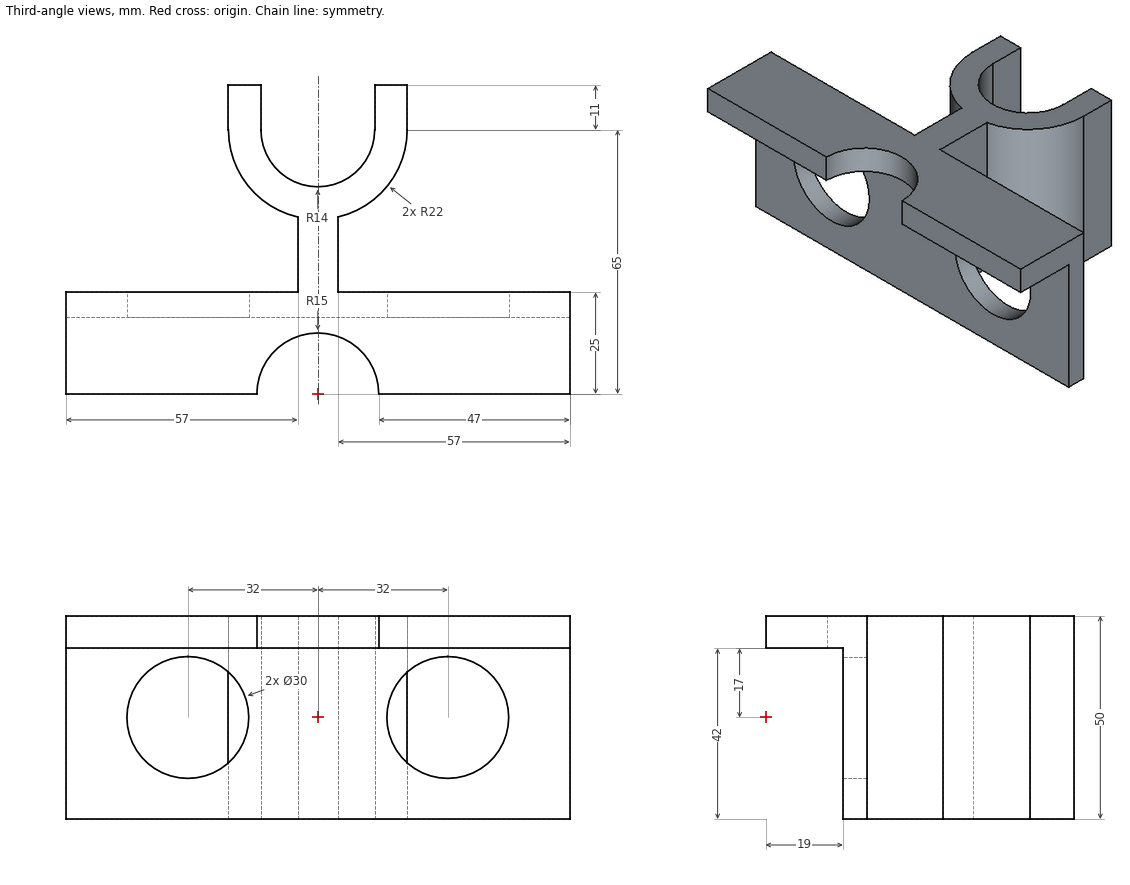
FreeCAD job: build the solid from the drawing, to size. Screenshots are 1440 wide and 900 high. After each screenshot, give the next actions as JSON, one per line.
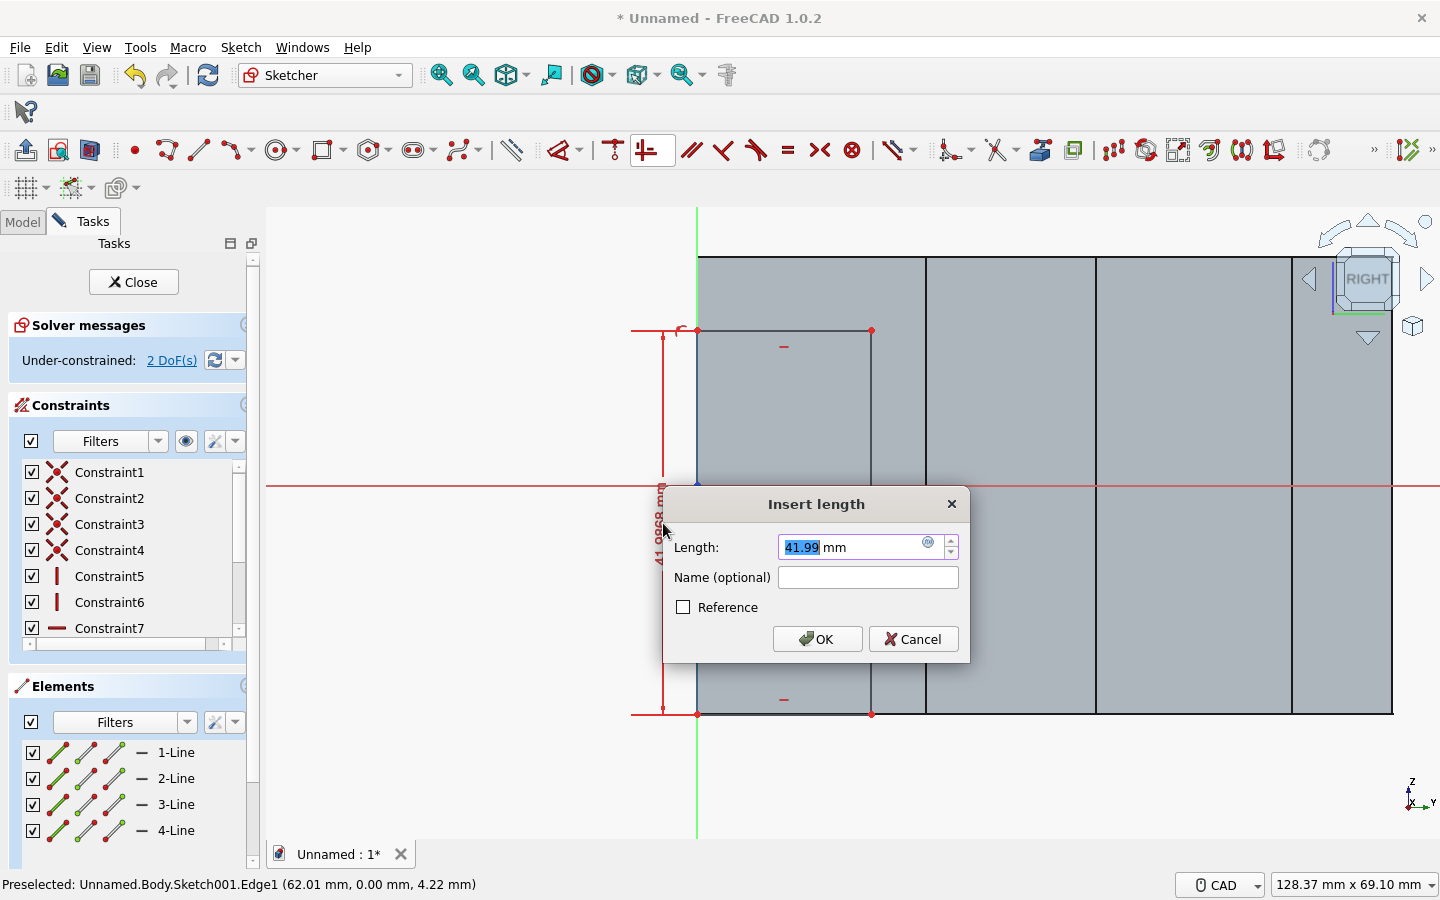
{"action": "type", "text": "42"}
{"action": "key", "text": "Return"}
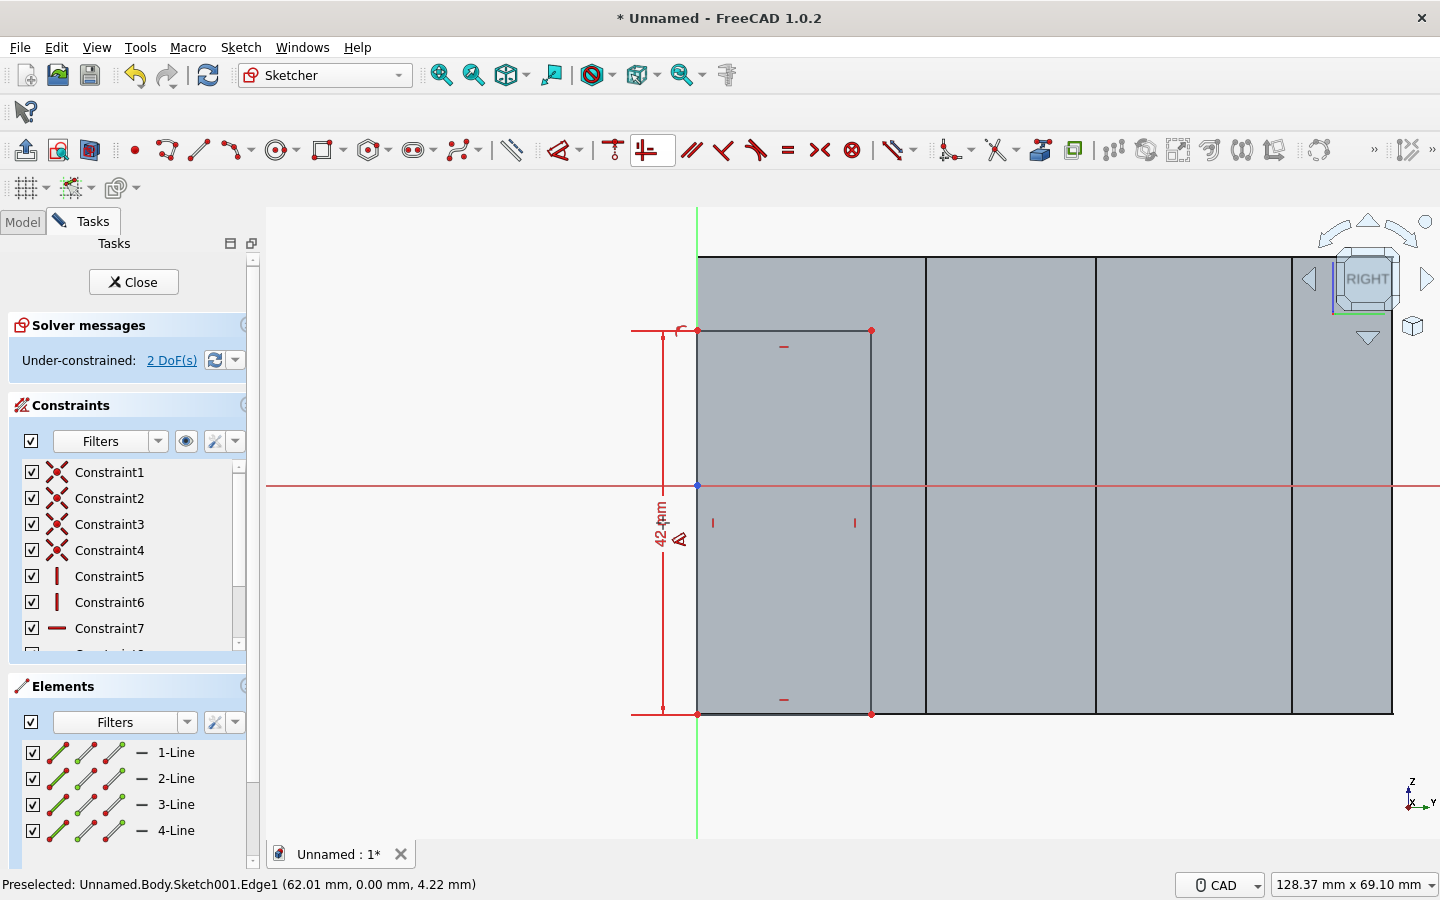
{"action": "left_click", "coordinate": [749, 715]}
{"action": "left_click", "coordinate": [784, 749]}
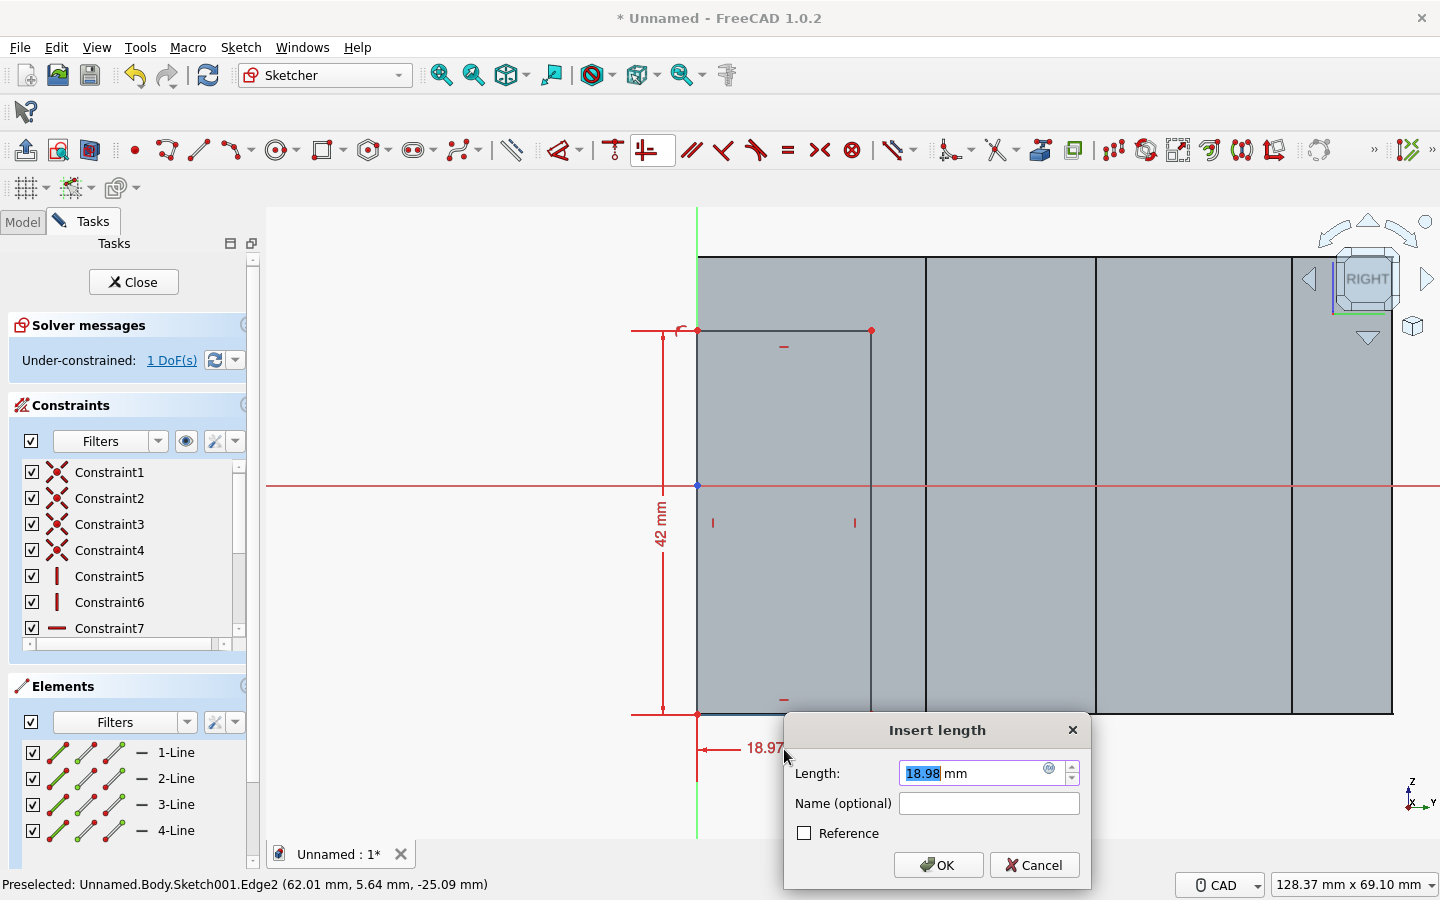
{"action": "type", "text": "19"}
{"action": "key", "text": "Return"}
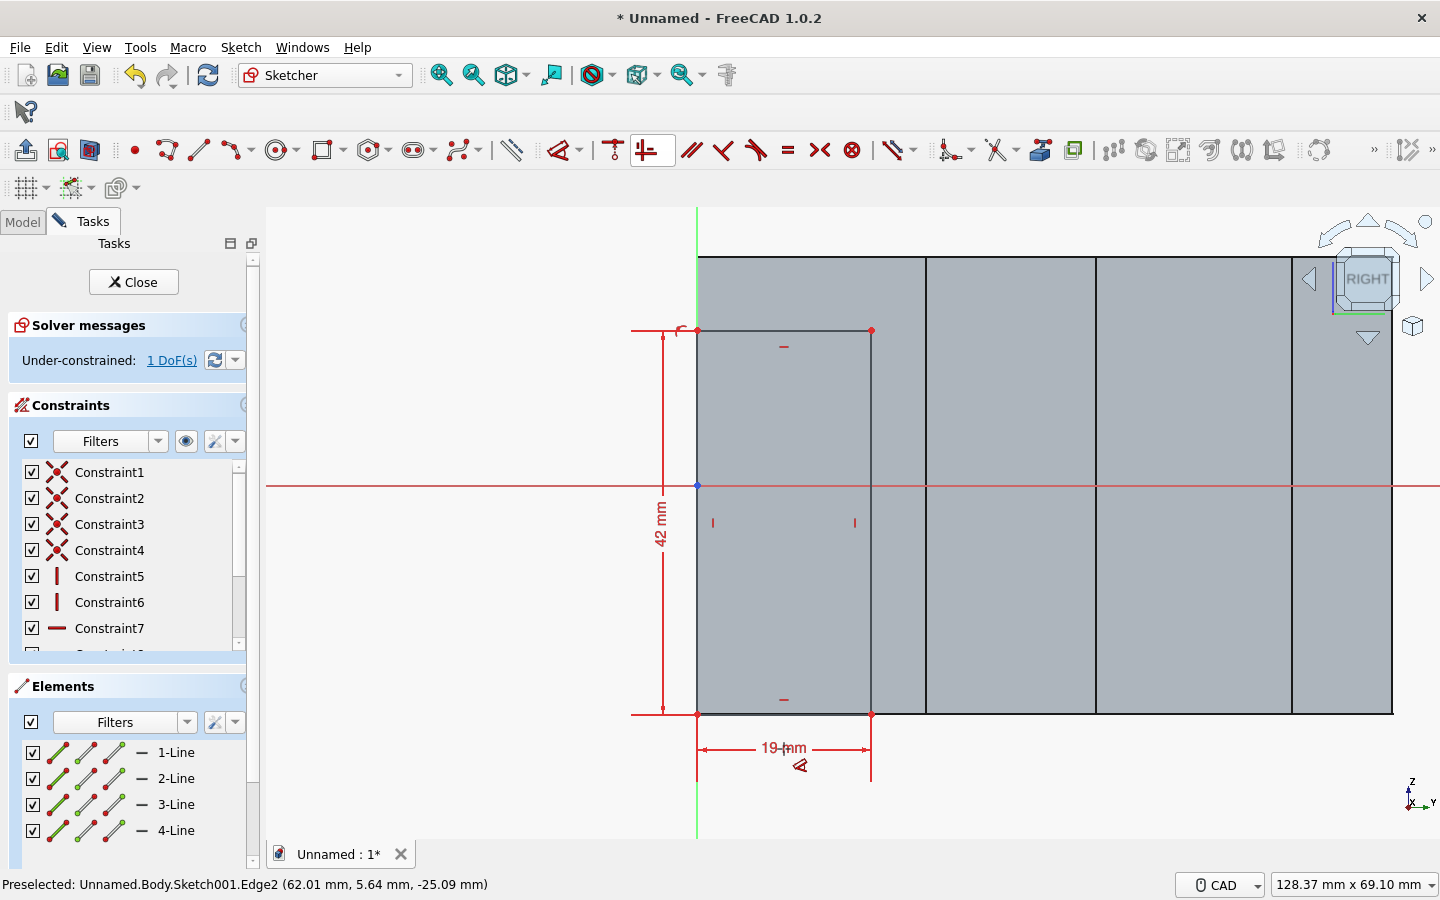
{"action": "left_click", "coordinate": [697, 331]}
{"action": "left_click", "coordinate": [663, 408]}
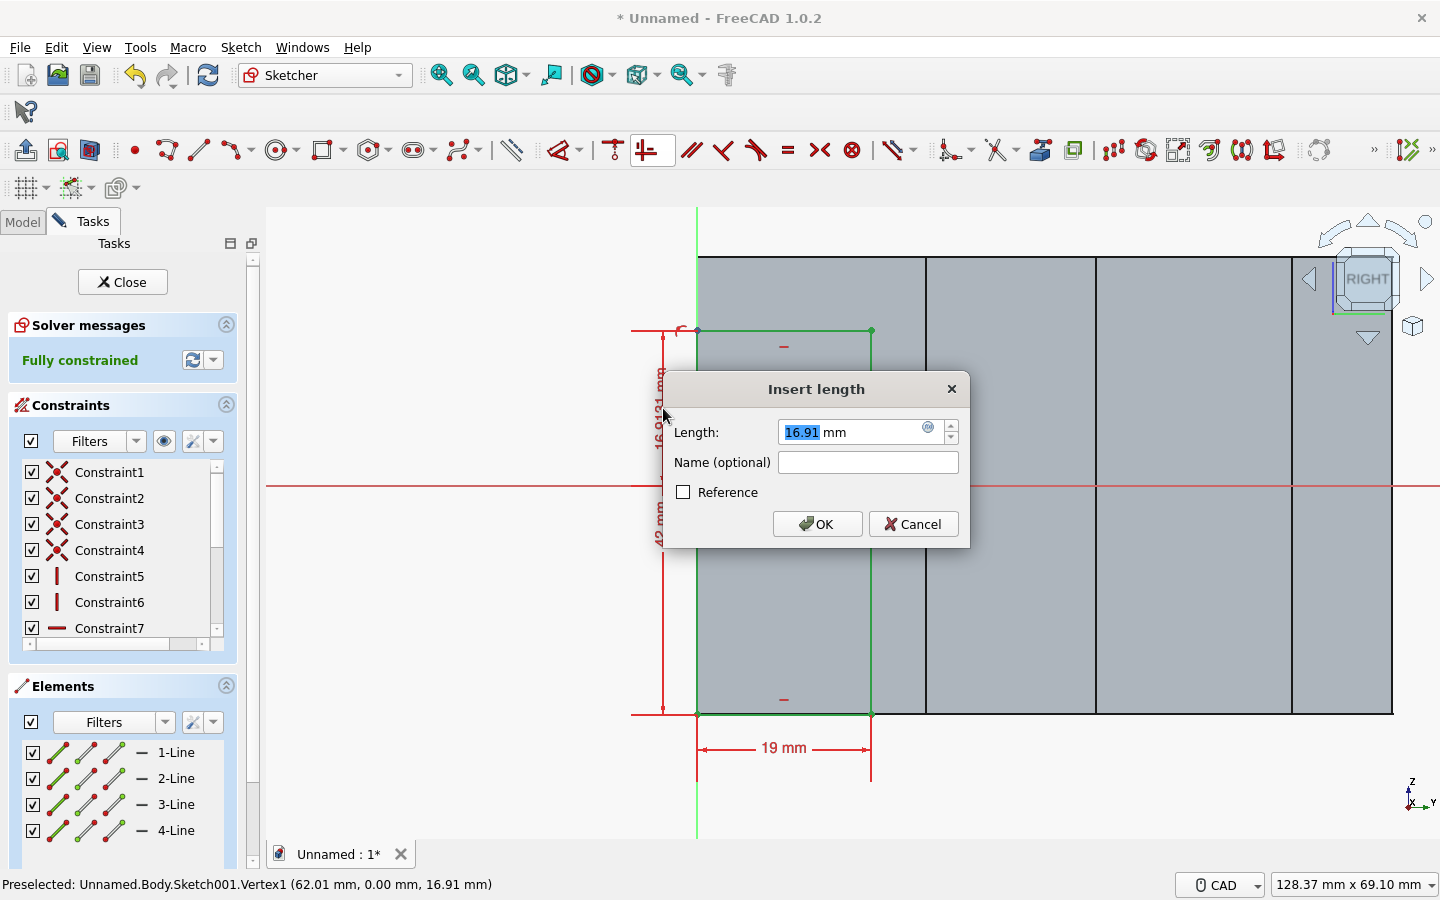
{"action": "type", "text": "17"}
{"action": "key", "text": "Return"}
{"action": "key", "text": "Escape"}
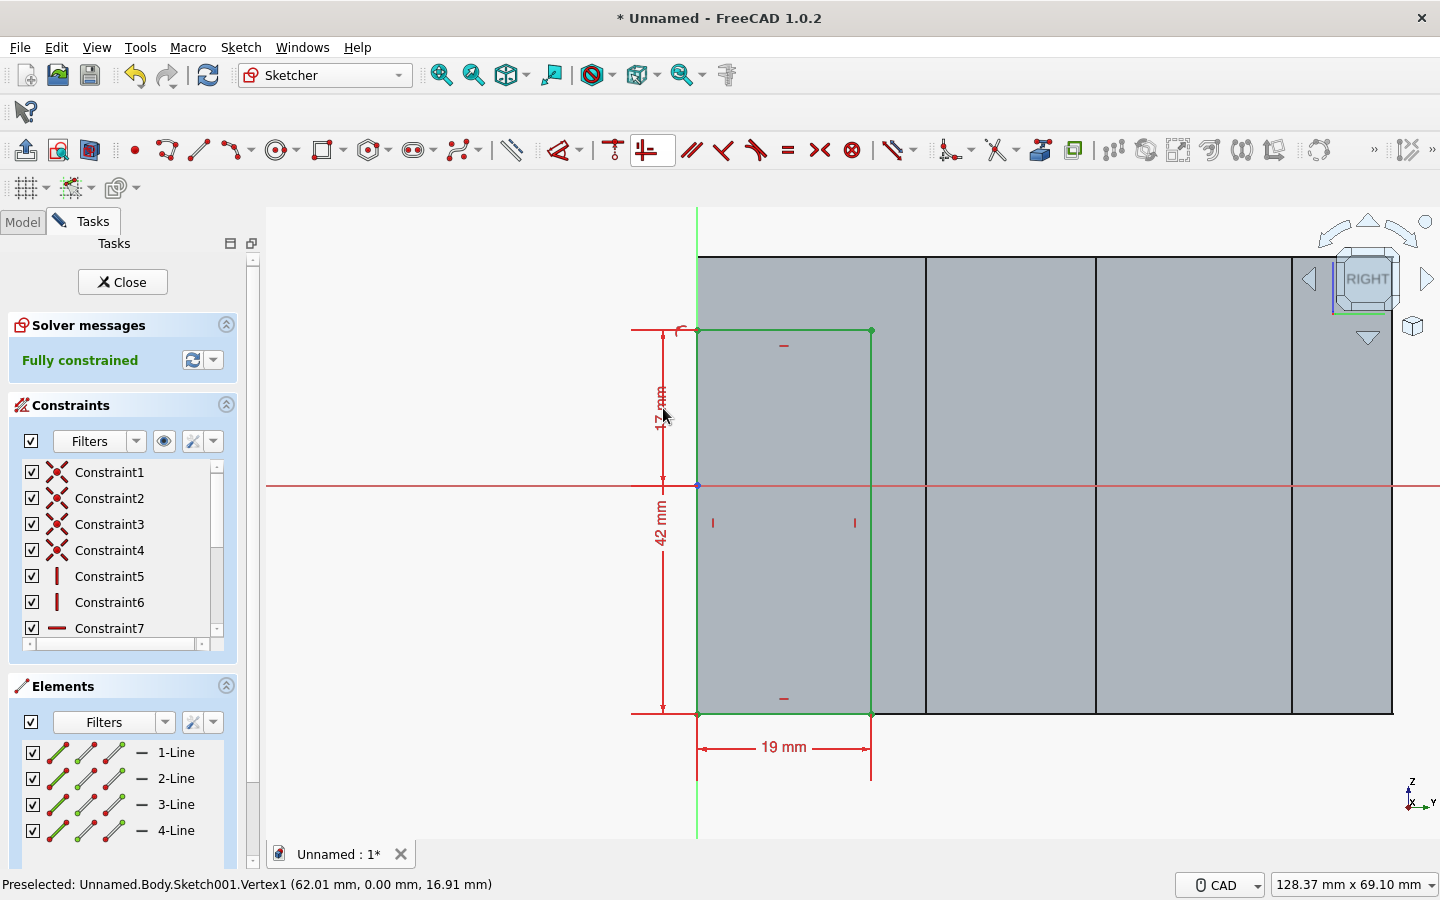
{"action": "left_click", "coordinate": [123, 282]}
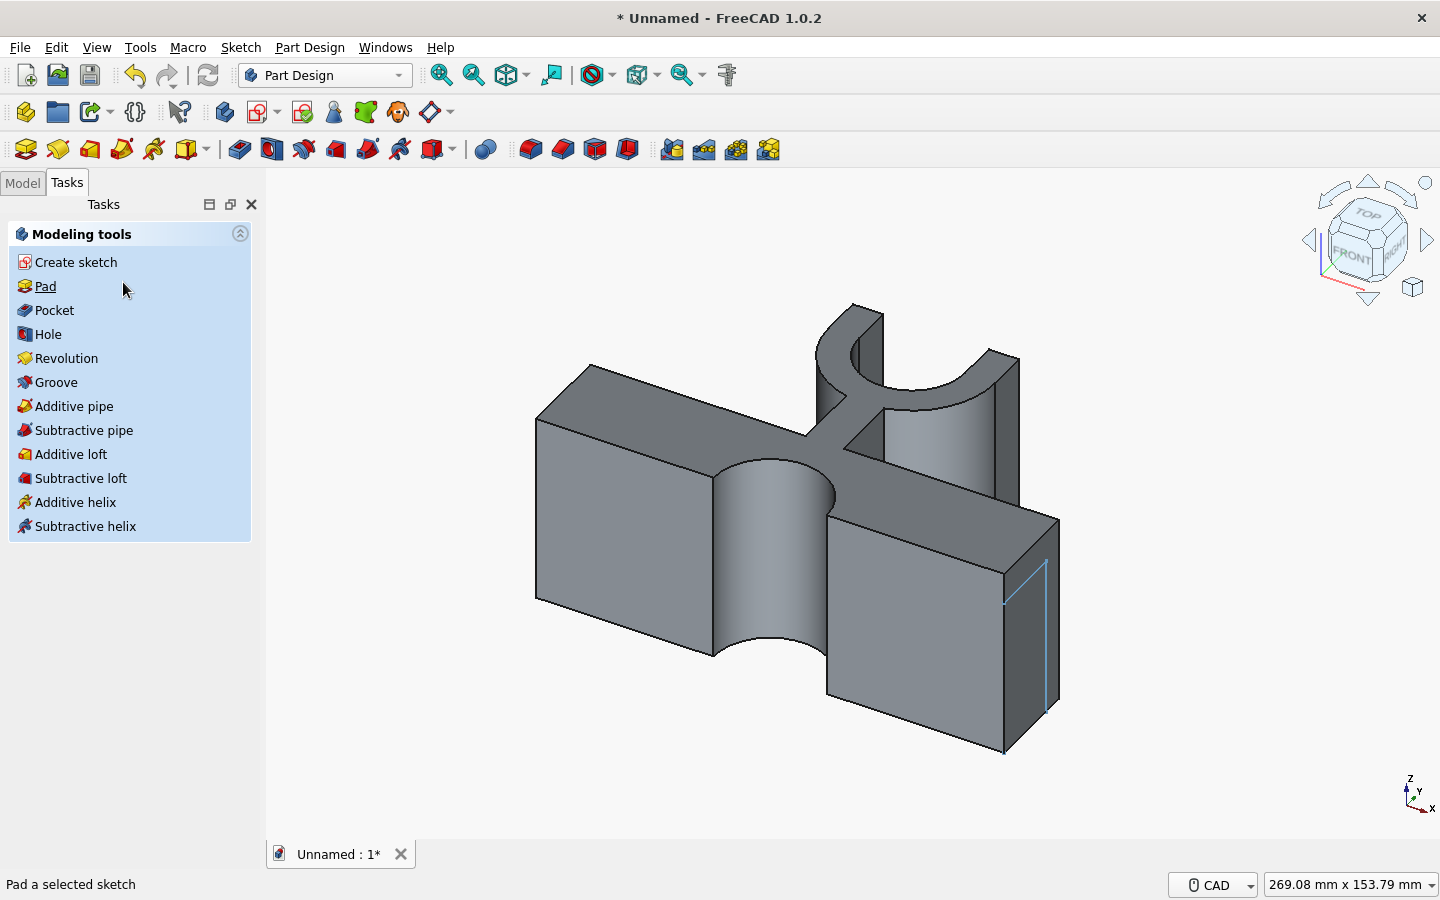
{"action": "left_click", "coordinate": [240, 150]}